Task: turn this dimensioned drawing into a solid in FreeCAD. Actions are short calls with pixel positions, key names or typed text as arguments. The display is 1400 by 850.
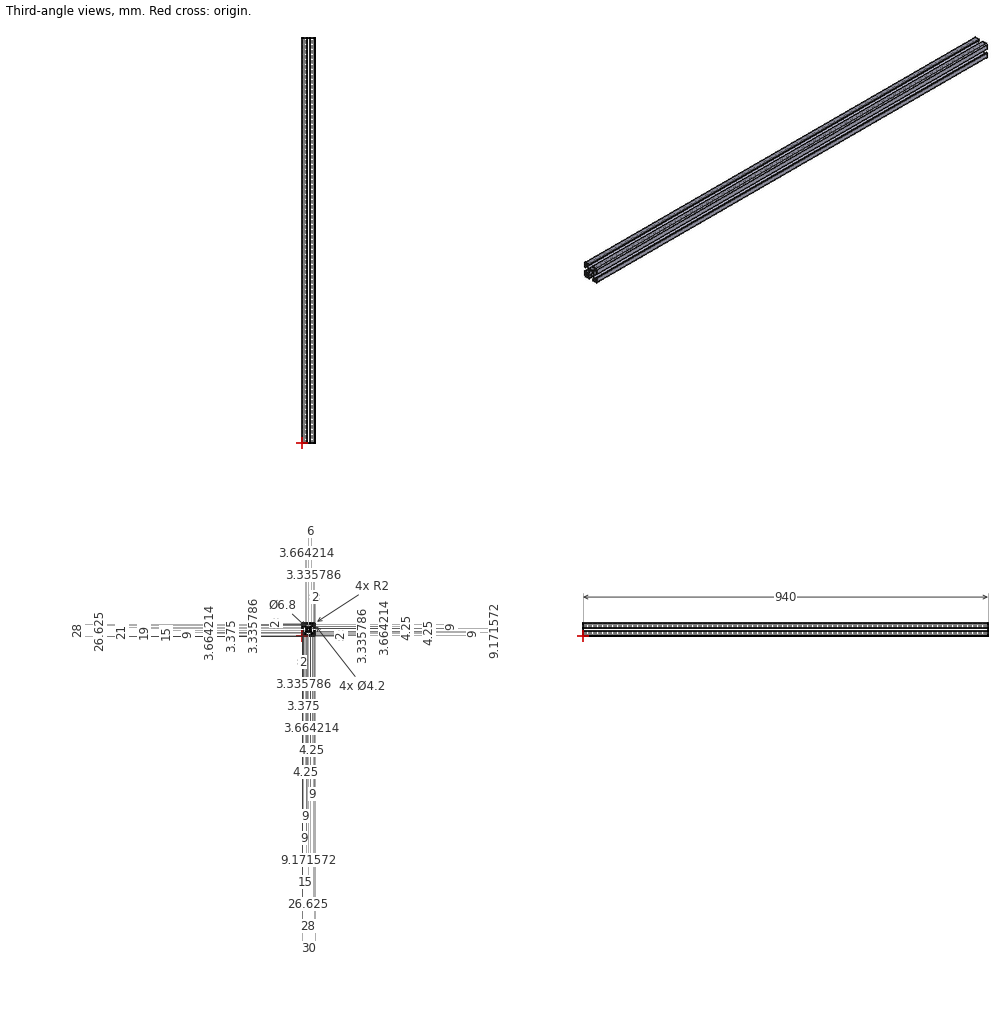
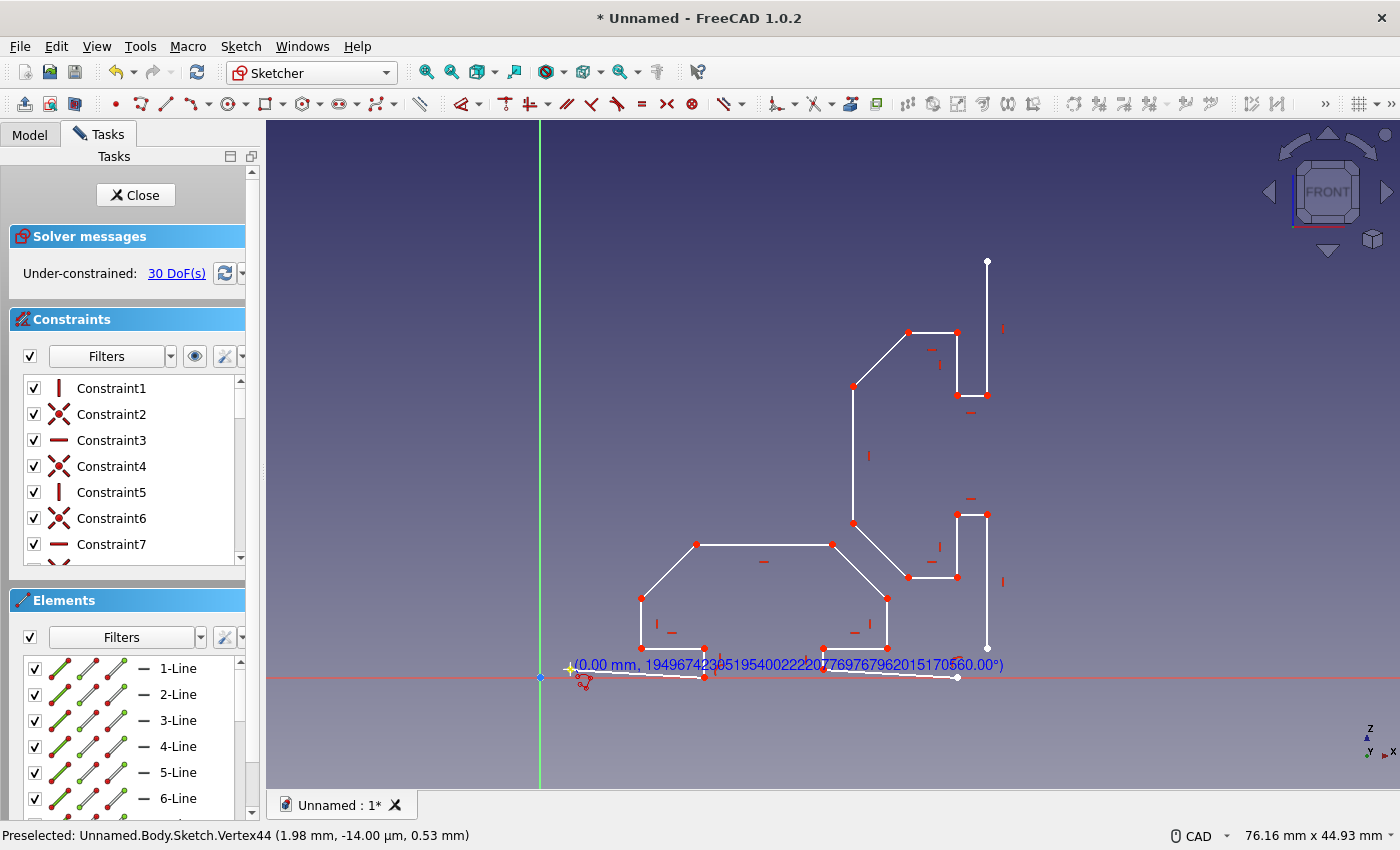
click(540, 648)
click(549, 514)
click(570, 514)
click(570, 577)
click(620, 577)
click(674, 523)
click(674, 386)
click(620, 332)
click(570, 332)
click(570, 395)
click(540, 395)
click(549, 261)
right_click(549, 261)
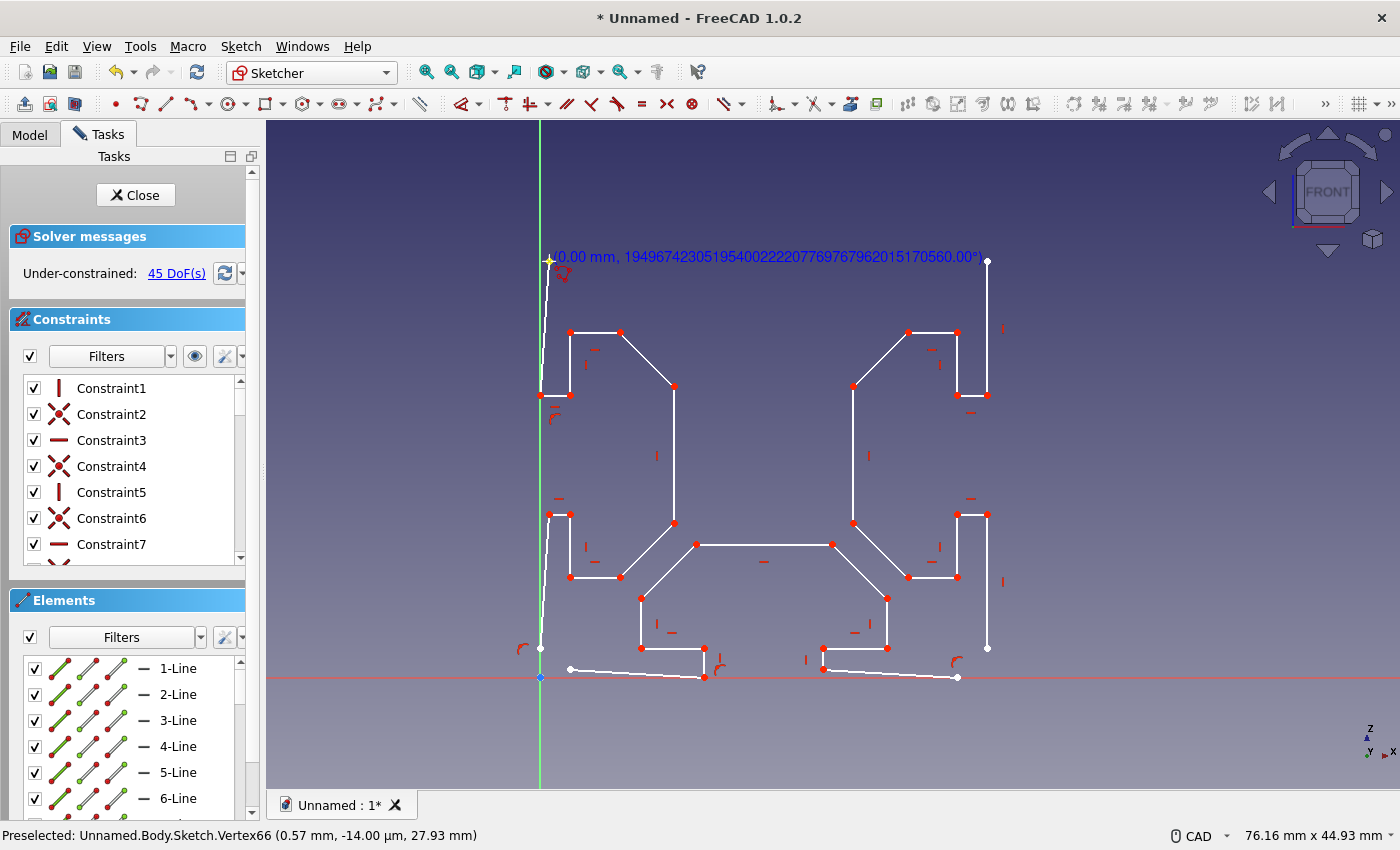
click(570, 231)
click(704, 231)
click(704, 261)
click(641, 261)
click(641, 311)
click(696, 365)
click(832, 365)
click(887, 311)
click(887, 261)
click(823, 261)
click(823, 231)
click(957, 231)
right_click(957, 231)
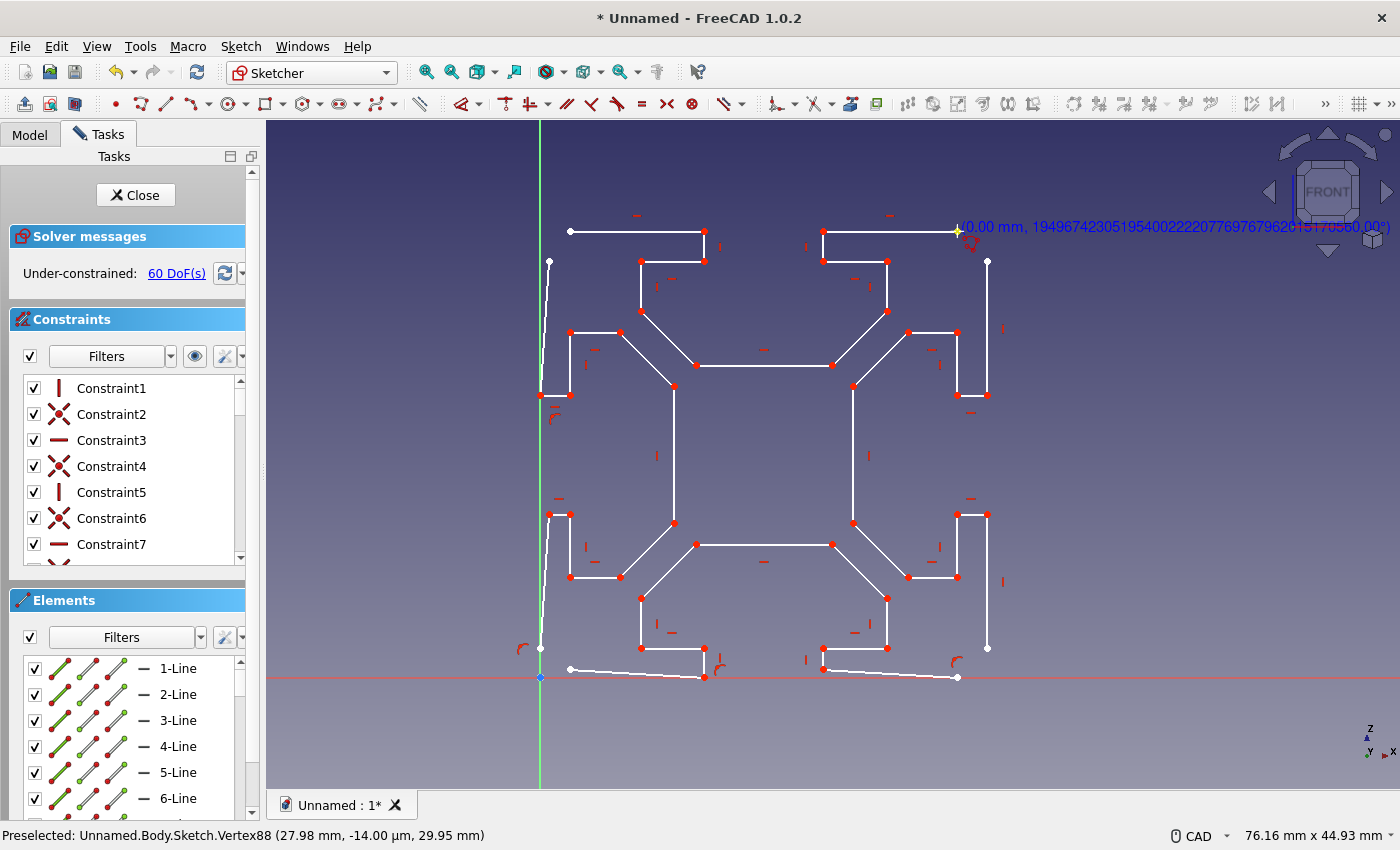
click(190, 104)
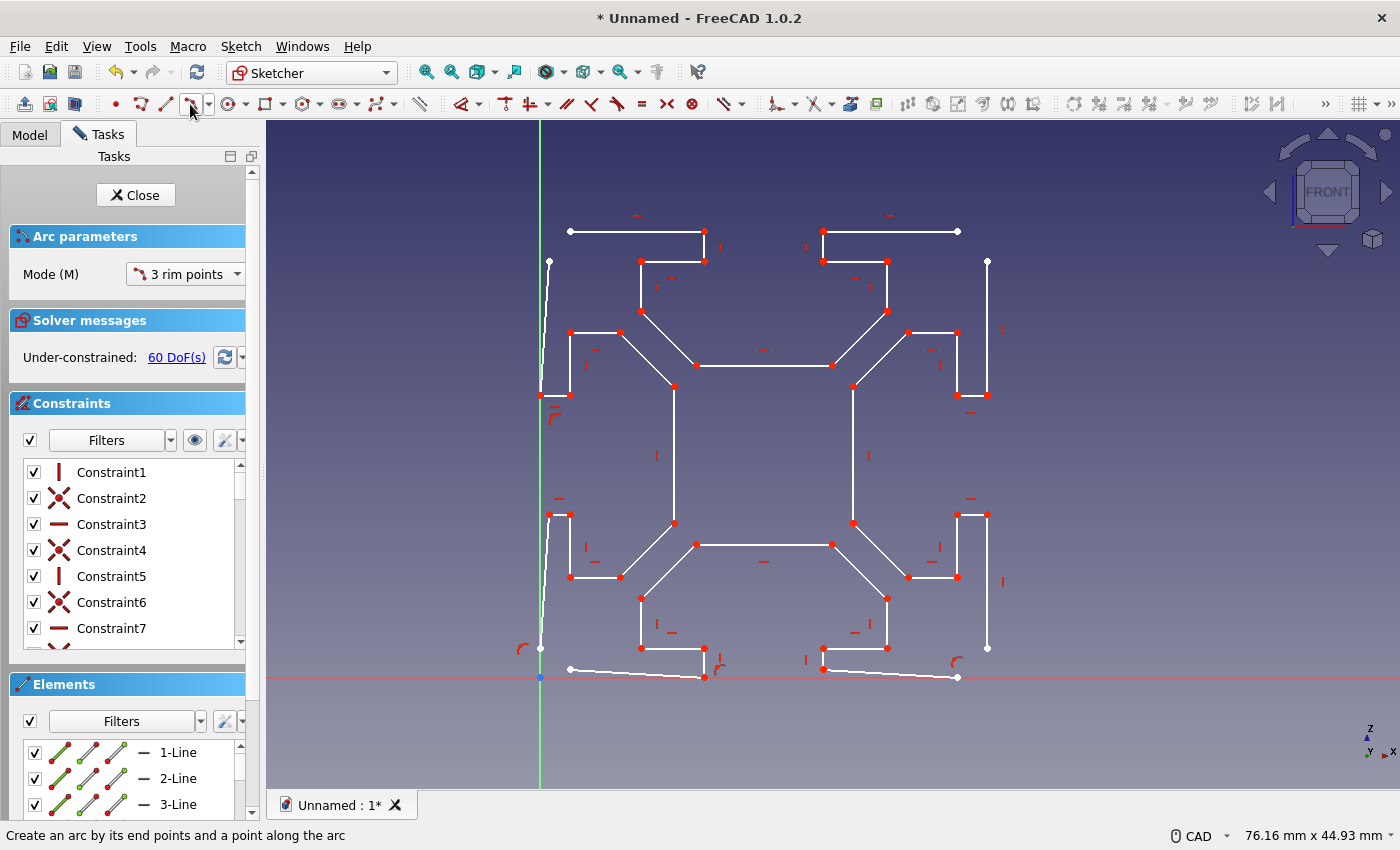
click(987, 649)
click(957, 678)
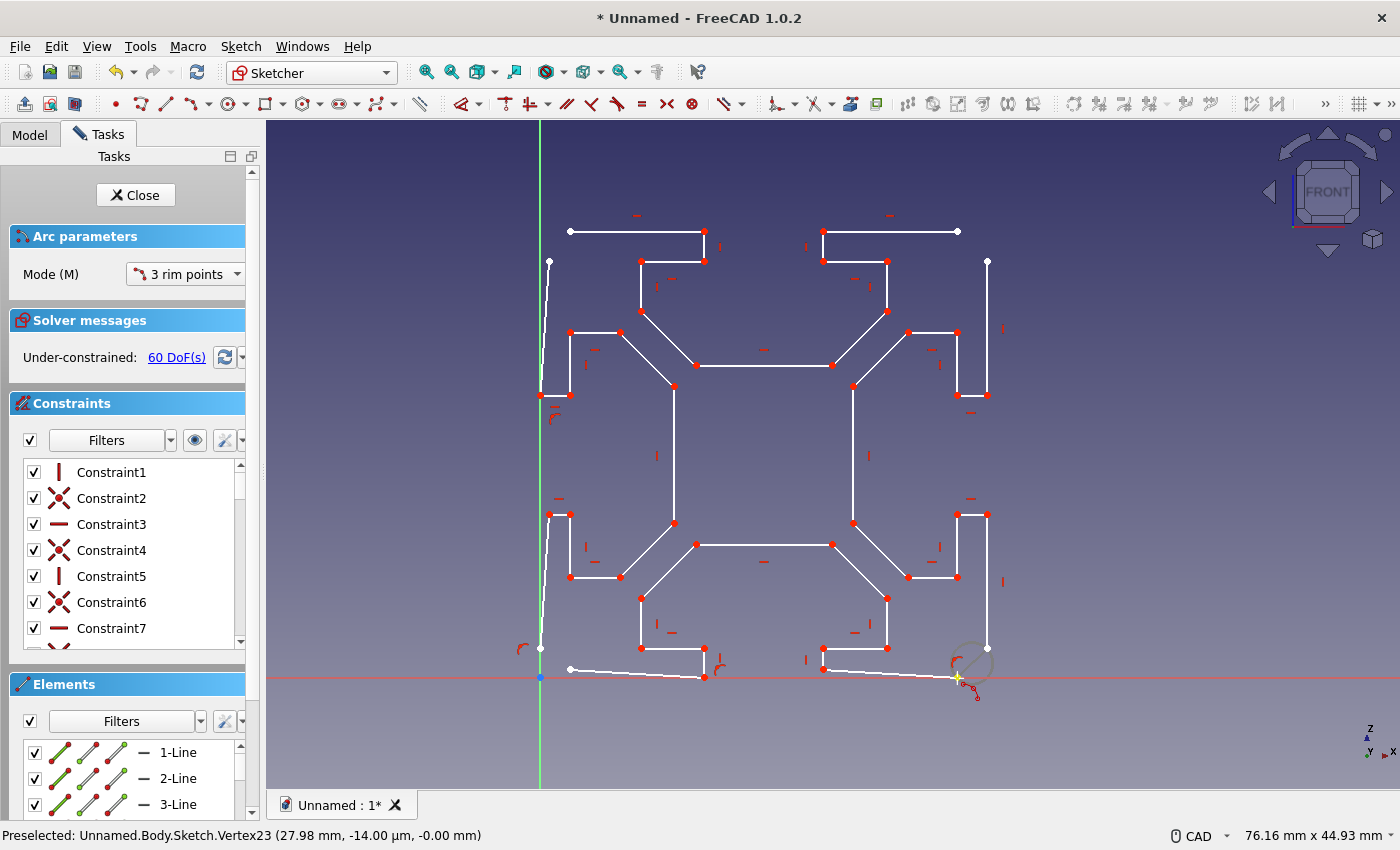
scroll(978, 669, up, 3)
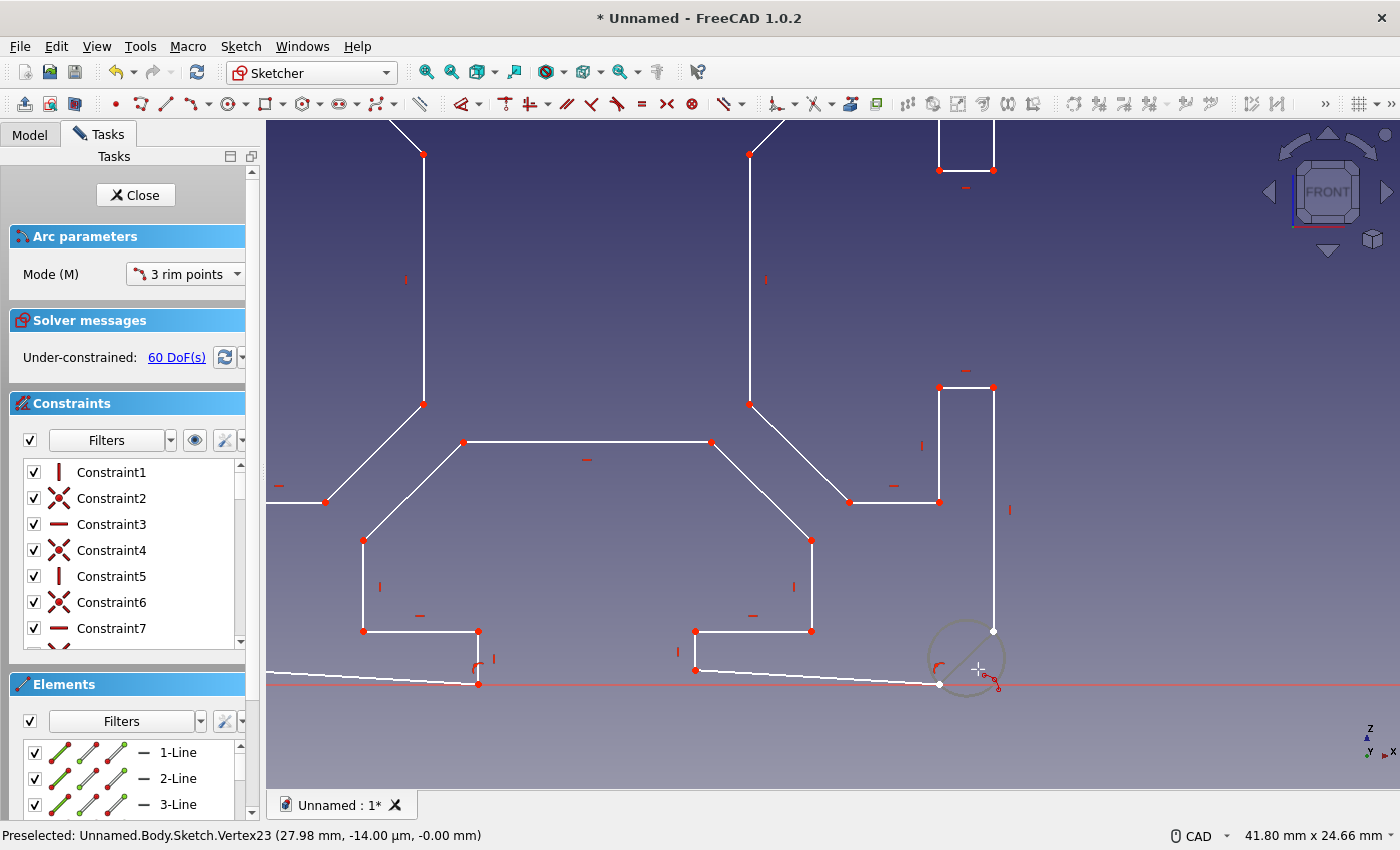
click(978, 669)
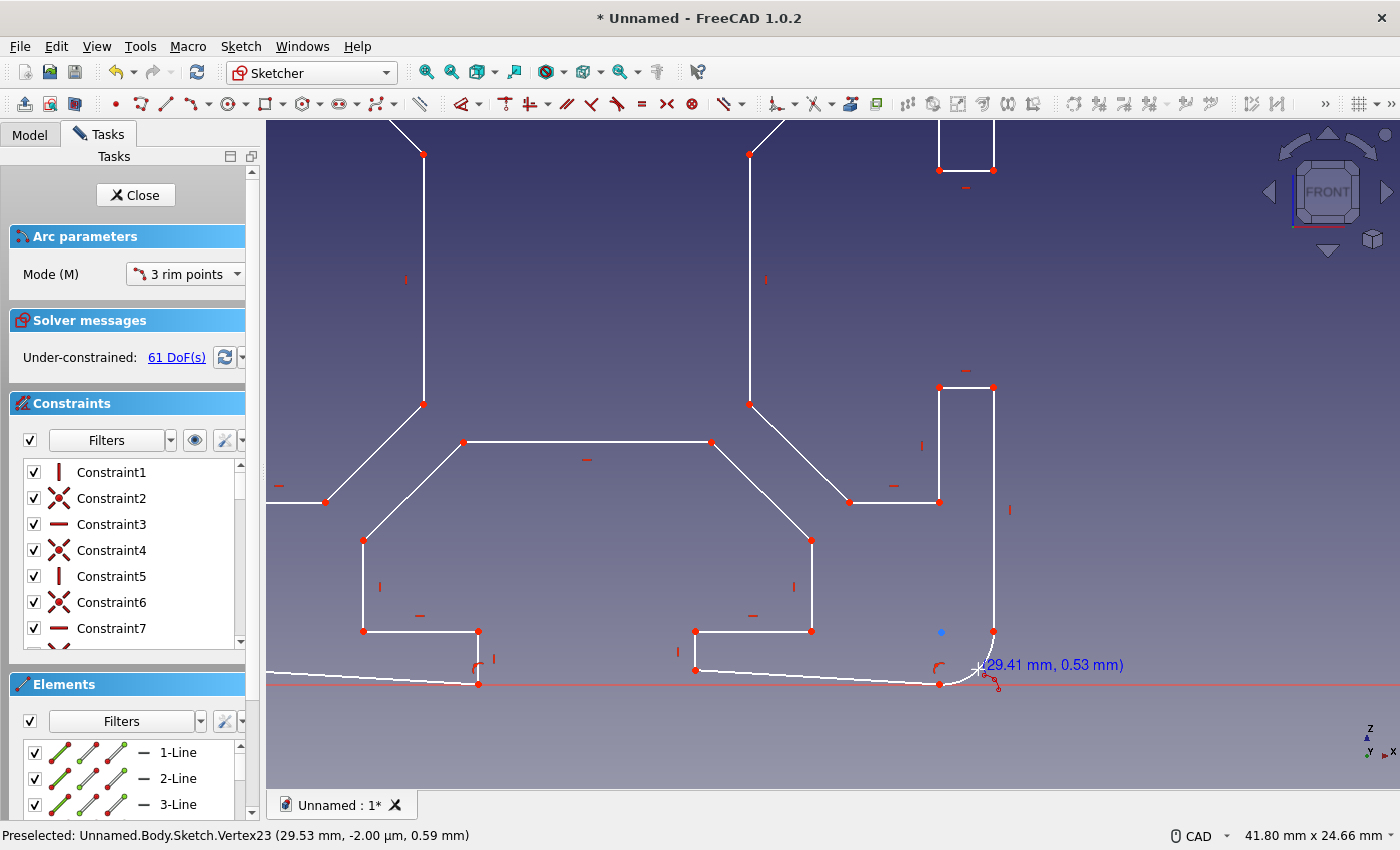
scroll(980, 670, down, 3)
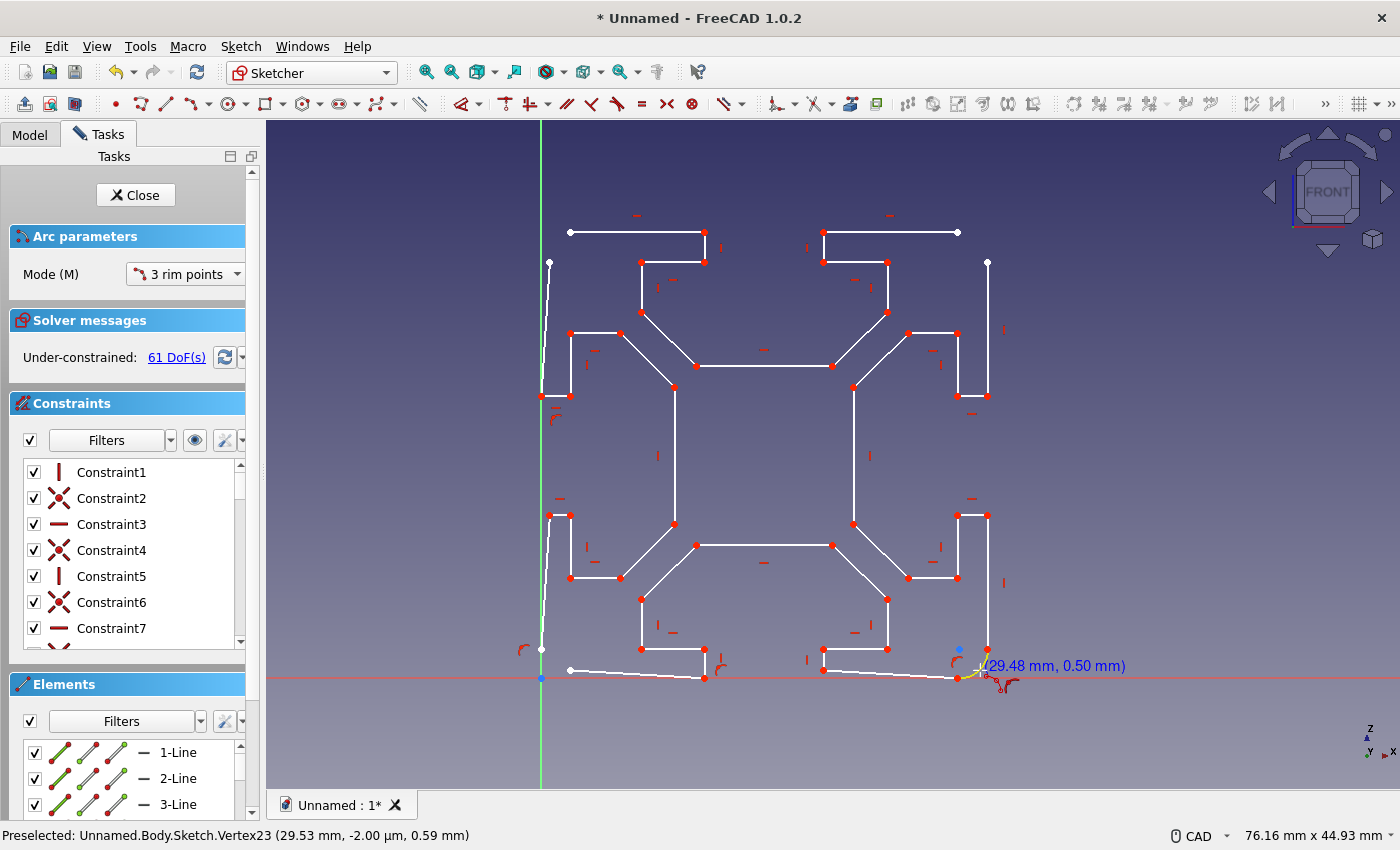
click(571, 670)
click(541, 649)